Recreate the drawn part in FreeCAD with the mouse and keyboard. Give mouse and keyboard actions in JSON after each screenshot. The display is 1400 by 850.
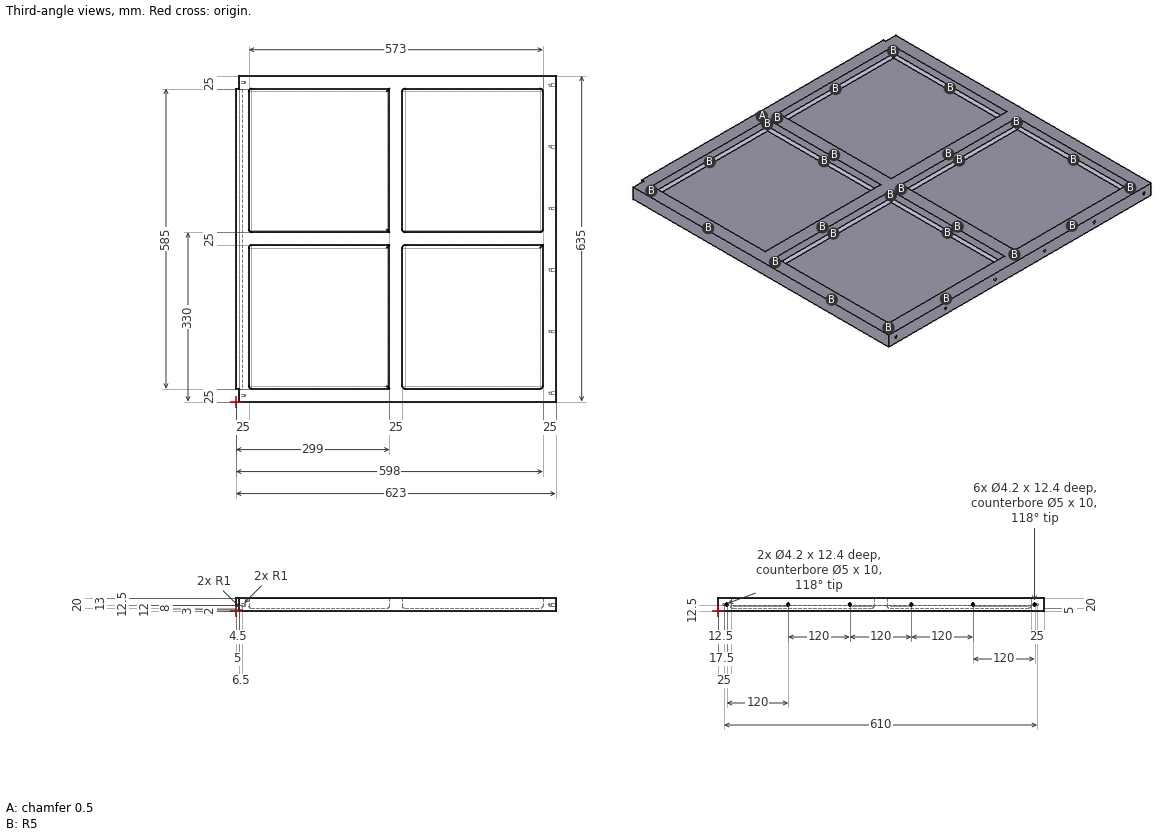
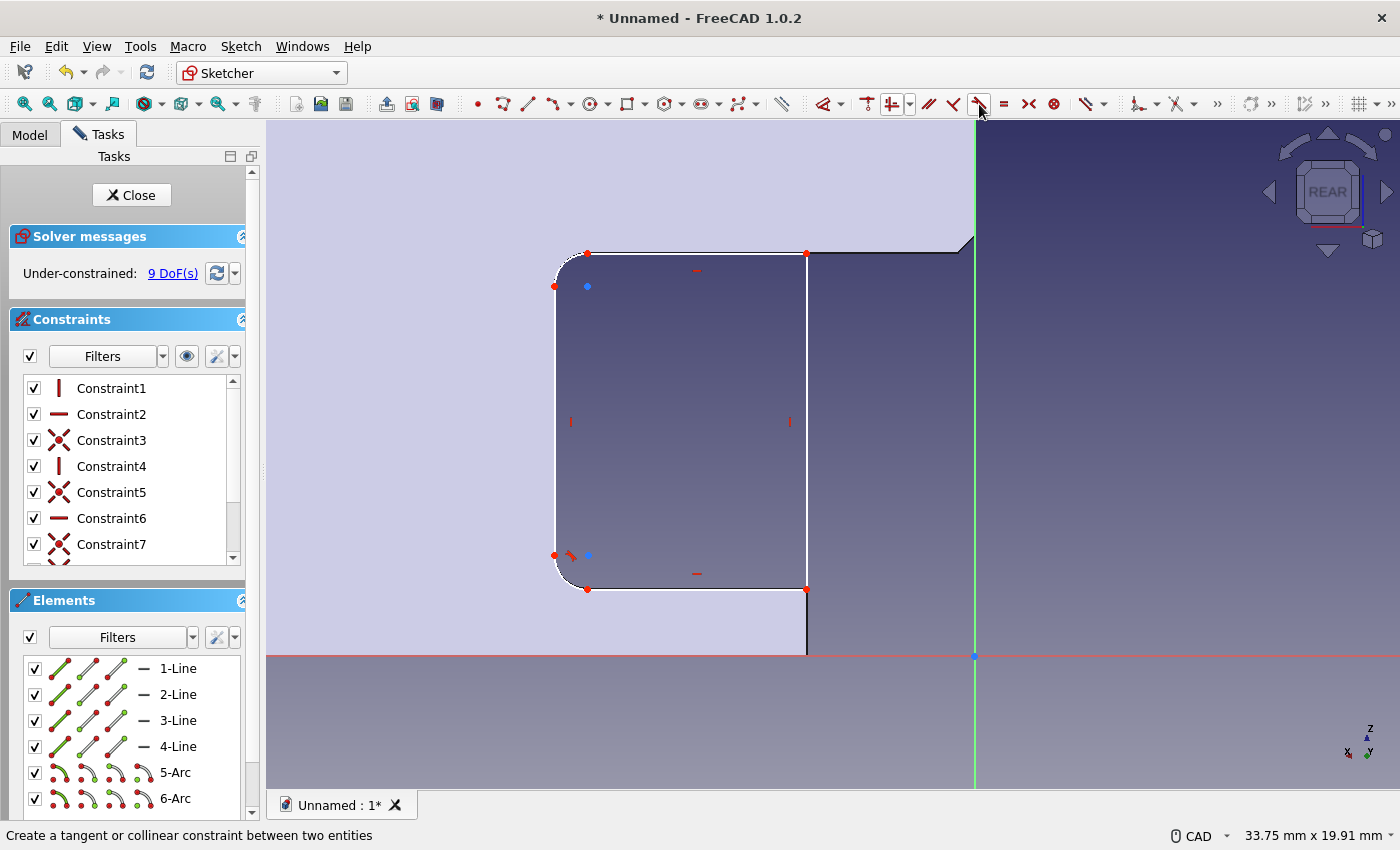
{"action": "left_click", "coordinate": [555, 368]}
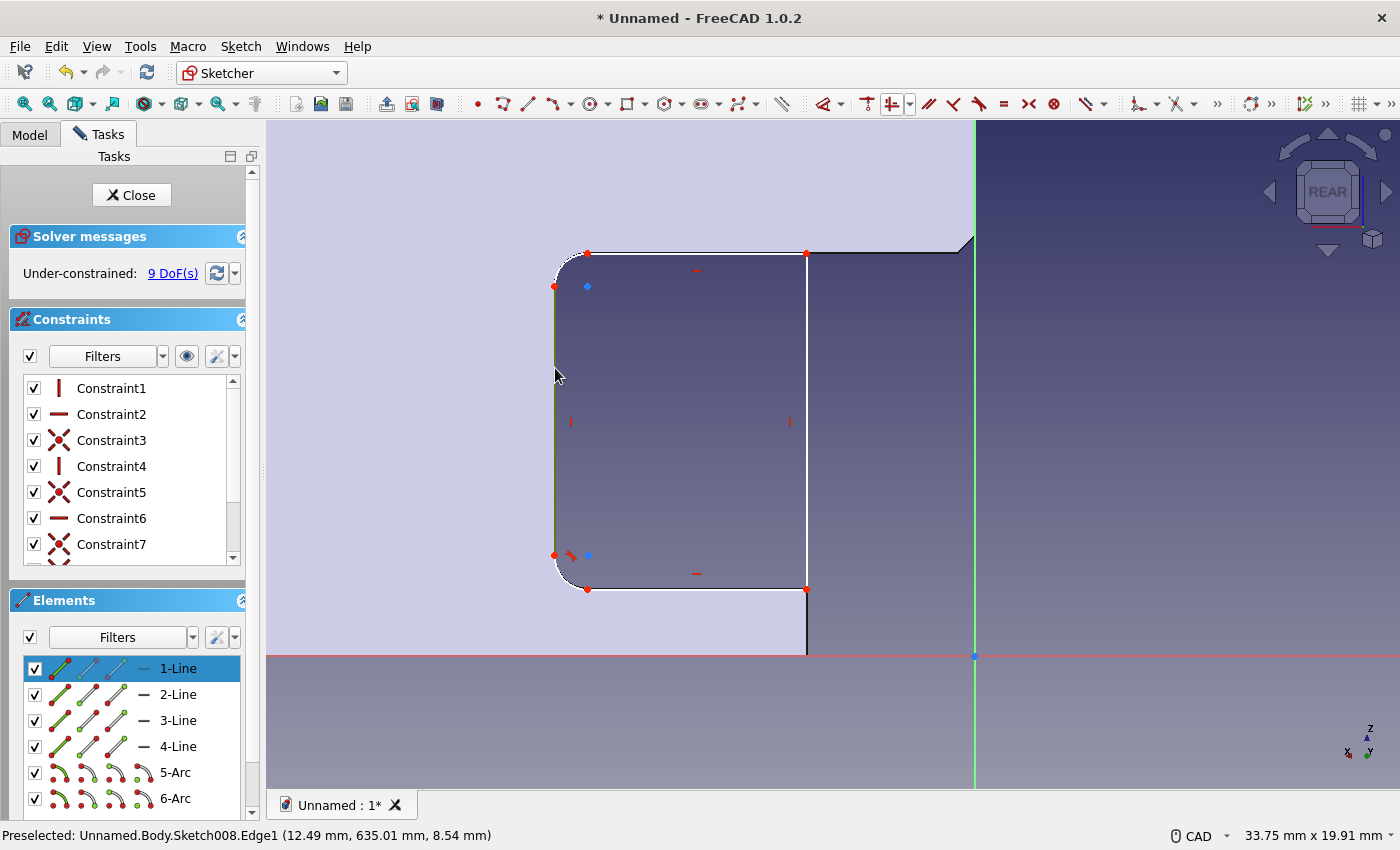
{"action": "left_click", "coordinate": [573, 257]}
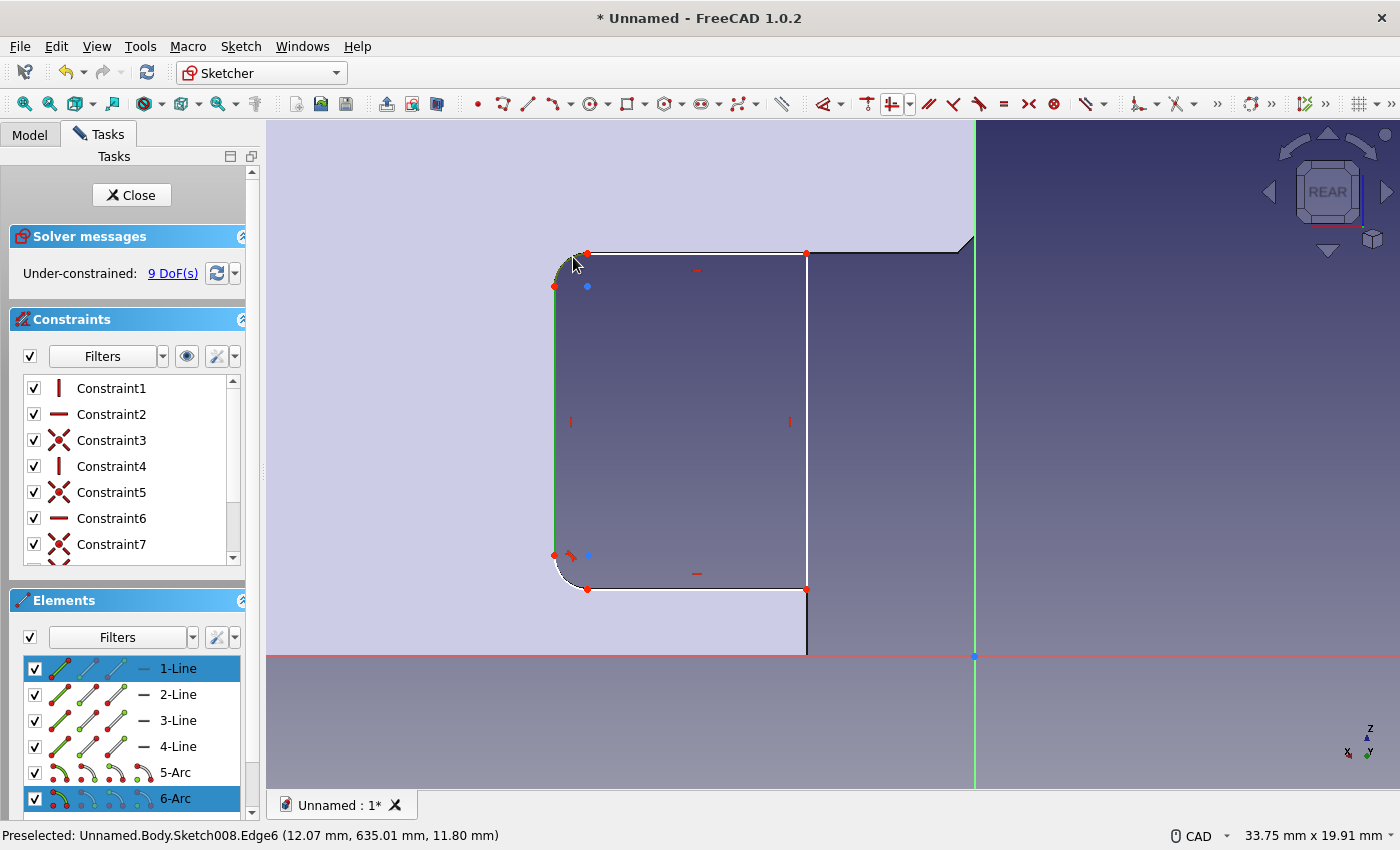
{"action": "left_click", "coordinate": [979, 104]}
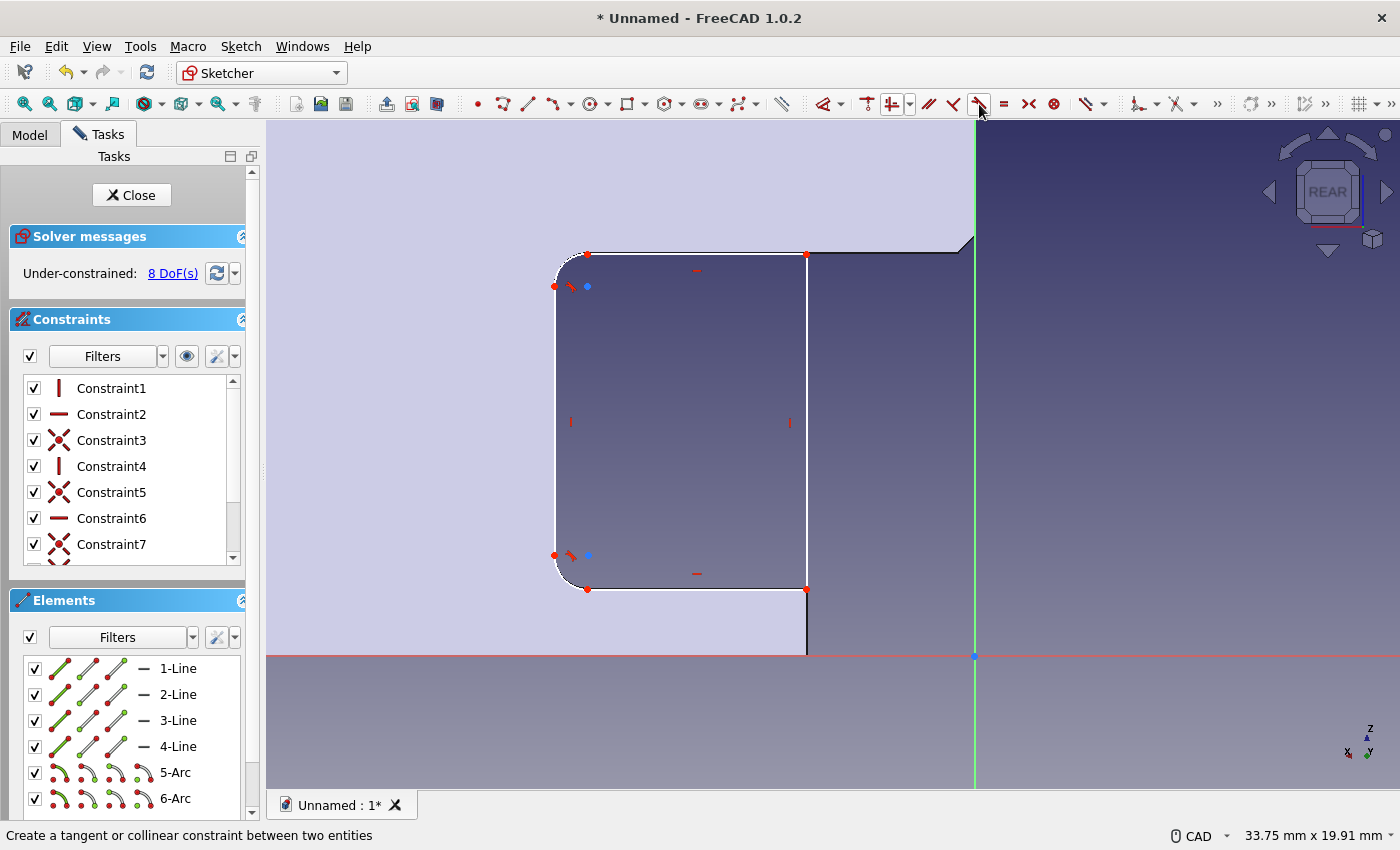
{"action": "left_click", "coordinate": [654, 590]}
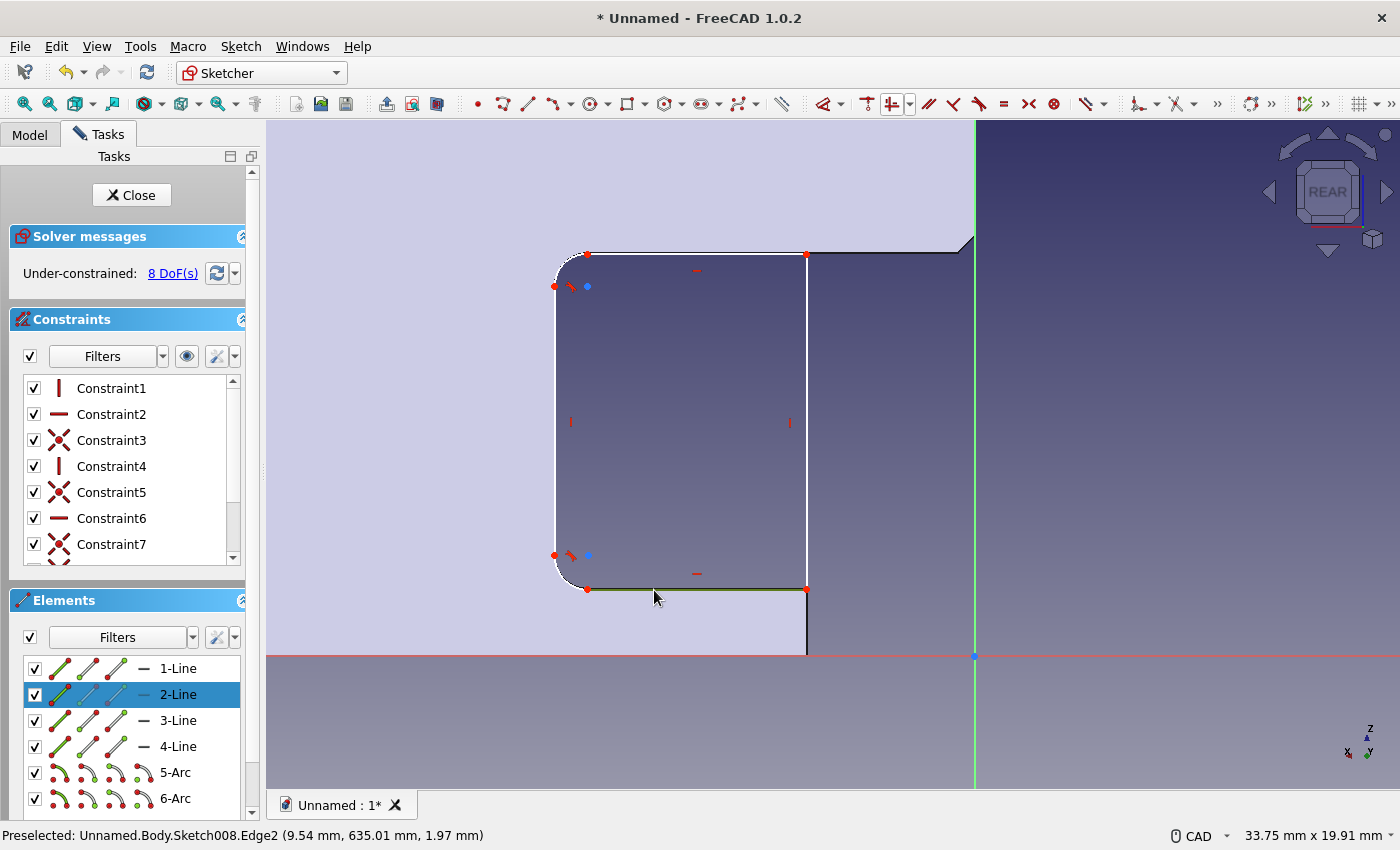
{"action": "left_click", "coordinate": [558, 571]}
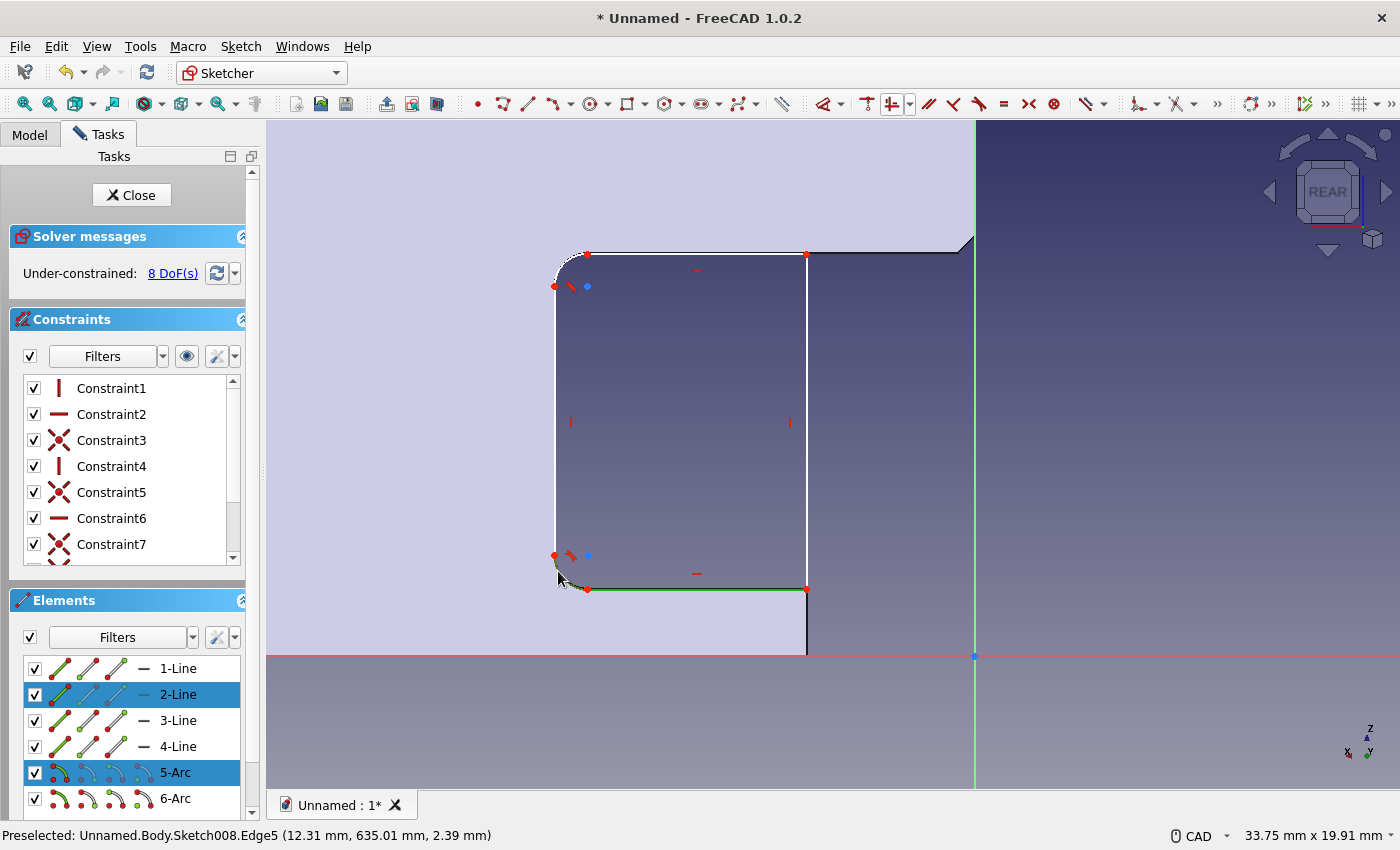
{"action": "left_click", "coordinate": [979, 104]}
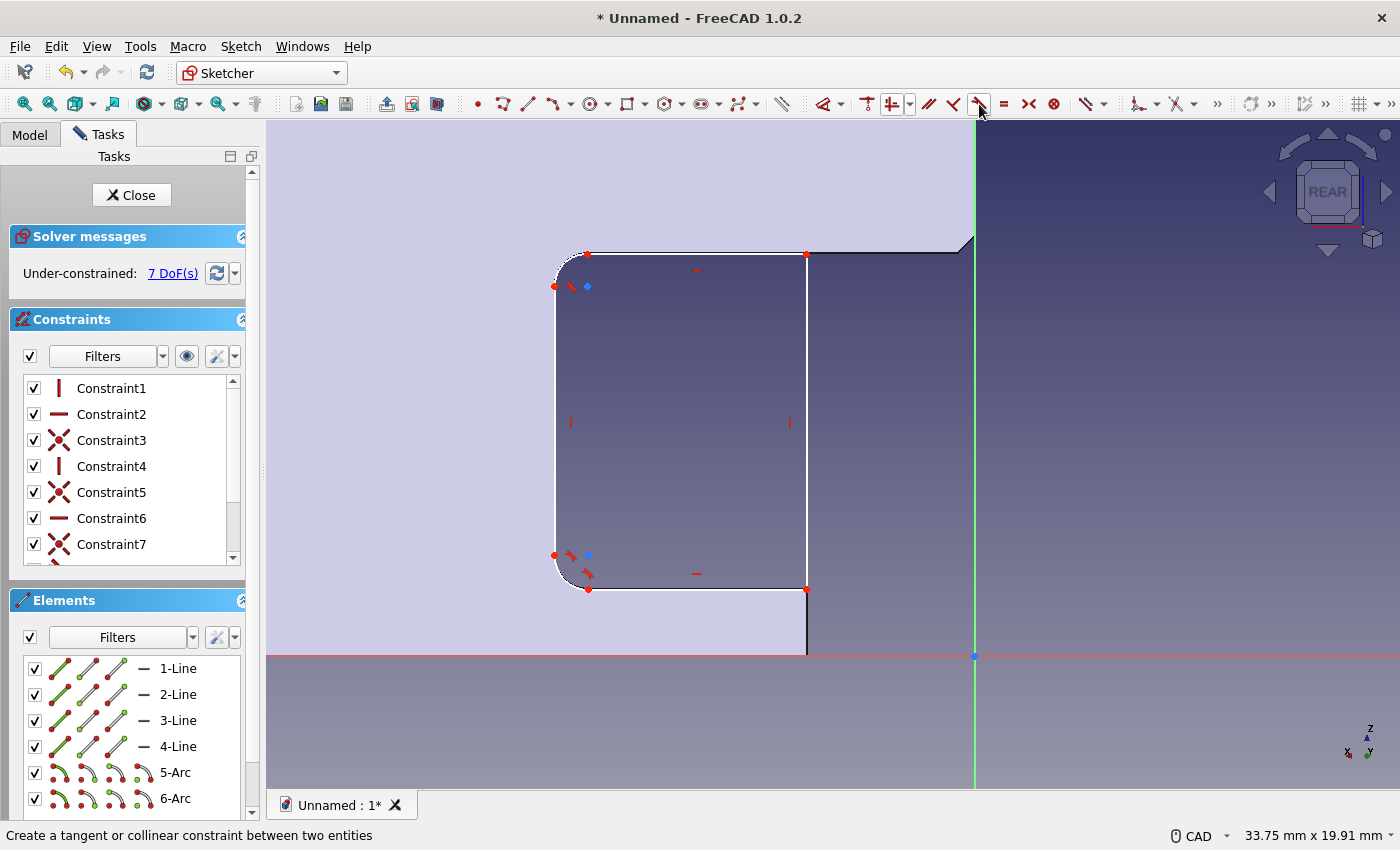
{"action": "left_click", "coordinate": [741, 254]}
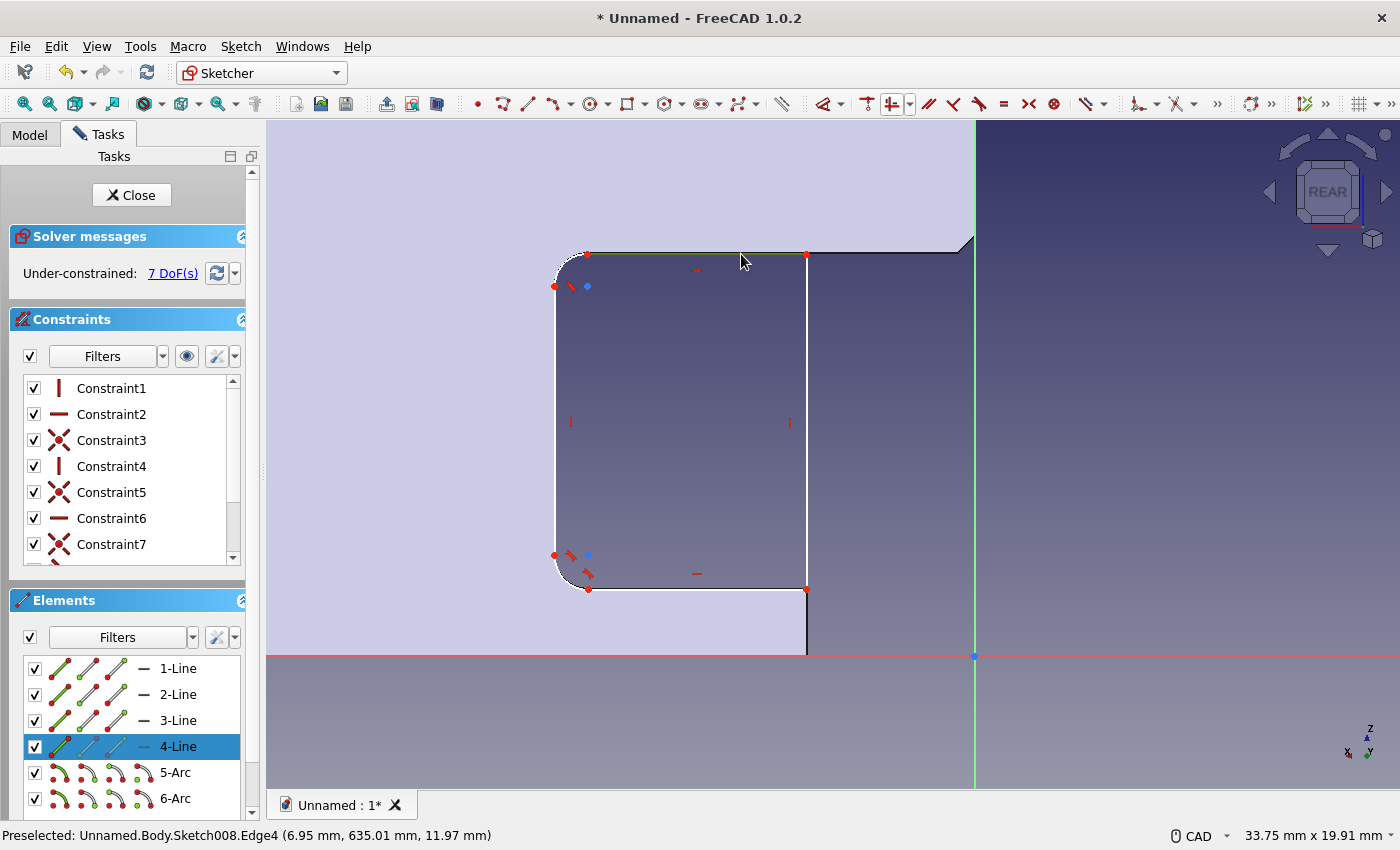
{"action": "left_click", "coordinate": [573, 257]}